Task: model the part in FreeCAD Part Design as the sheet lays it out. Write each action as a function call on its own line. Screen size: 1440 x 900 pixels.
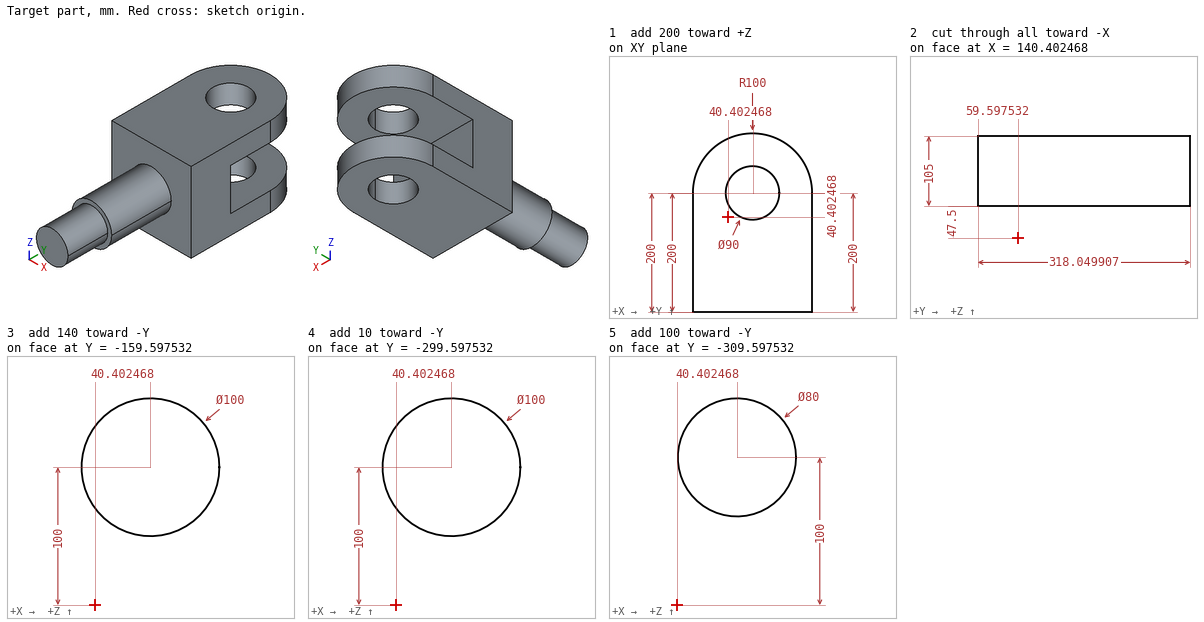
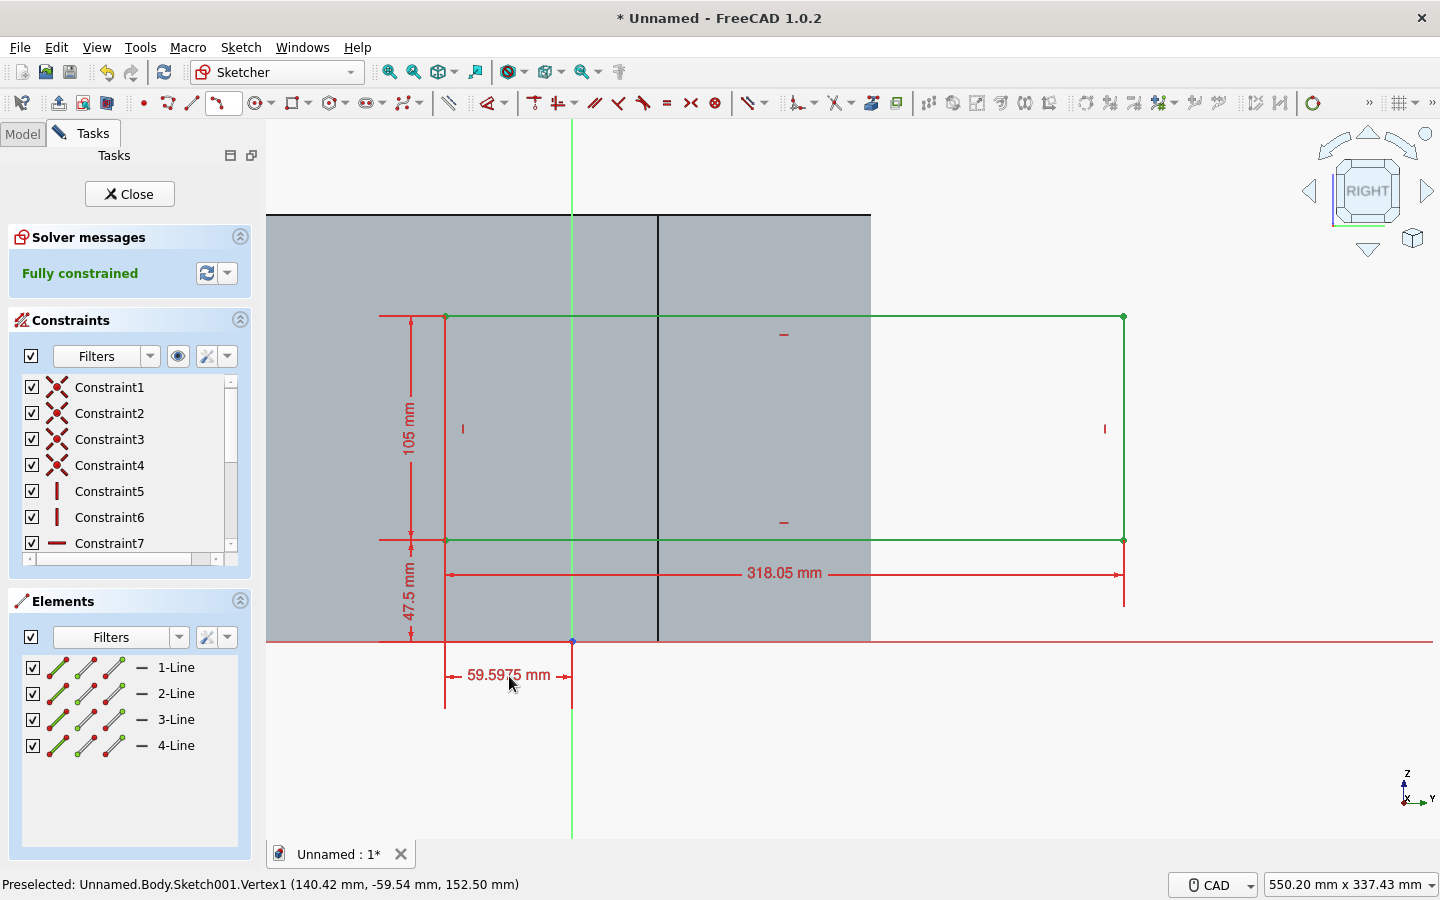
click(130, 194)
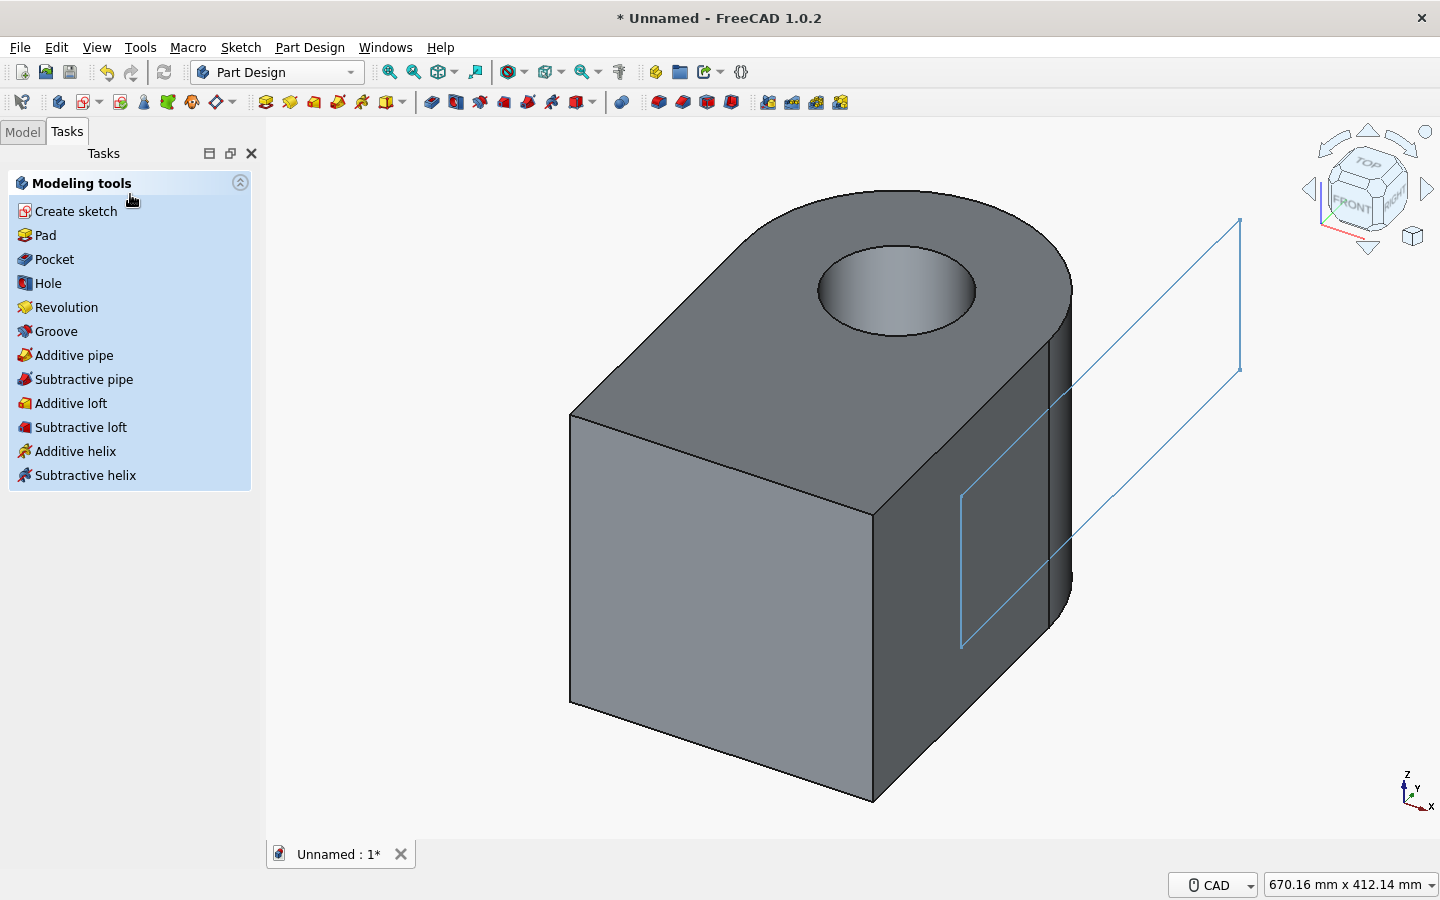
click(432, 102)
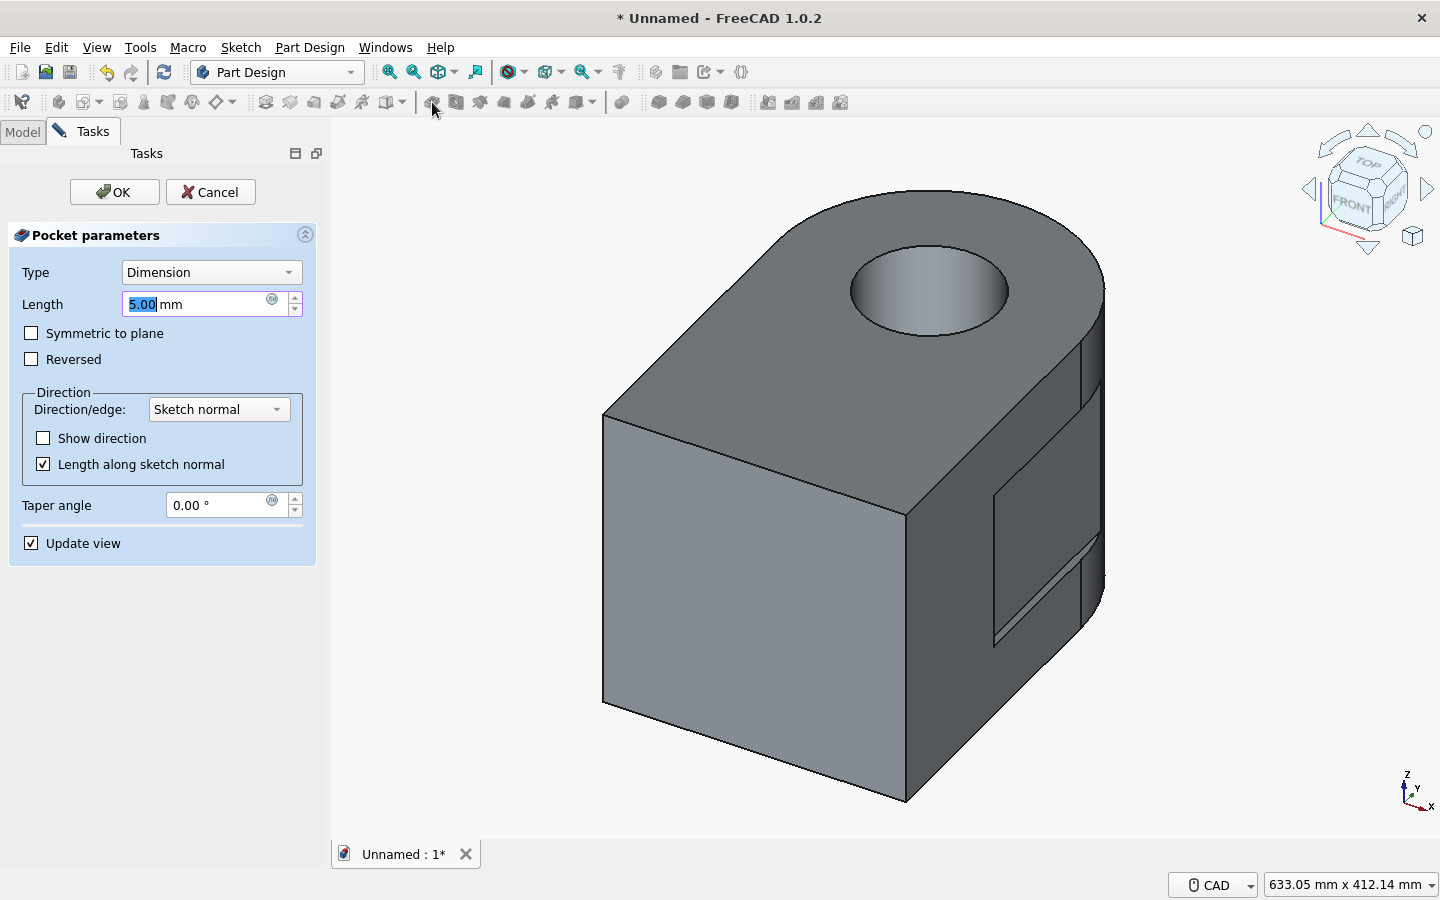
click(212, 272)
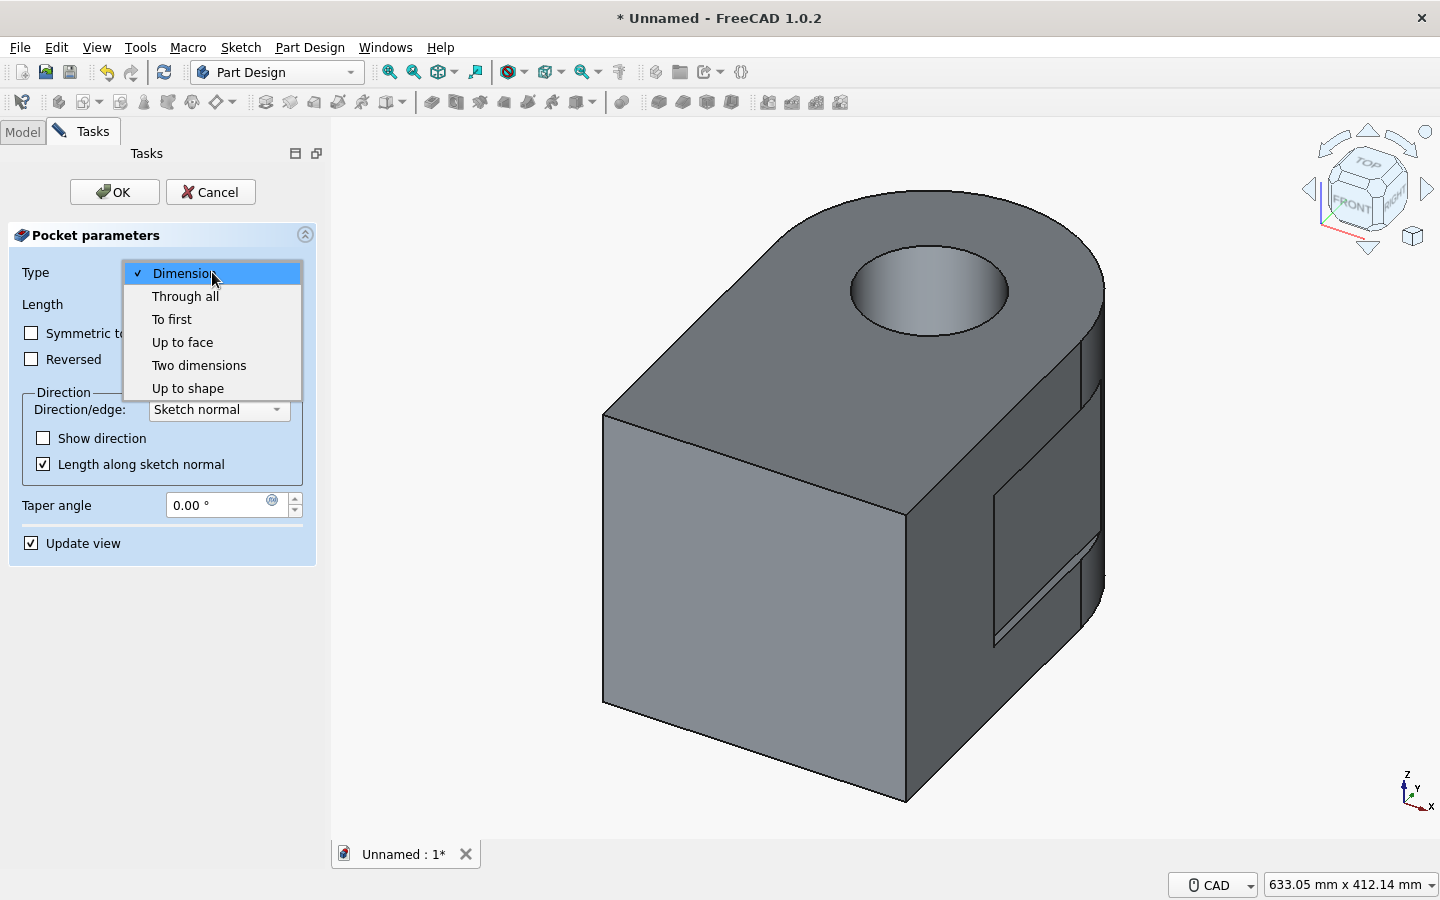
click(212, 296)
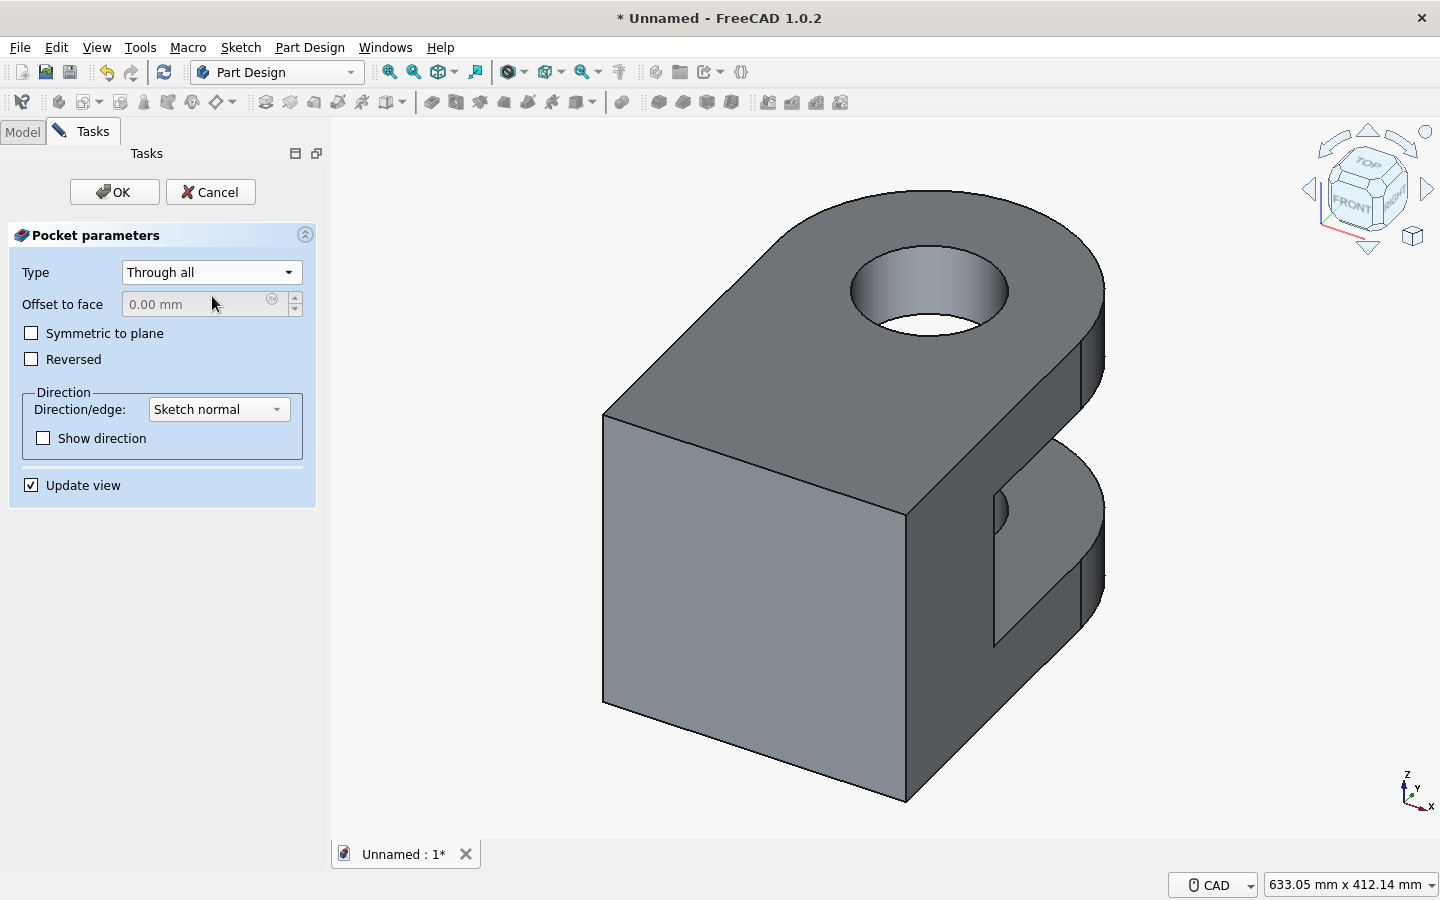
click(115, 192)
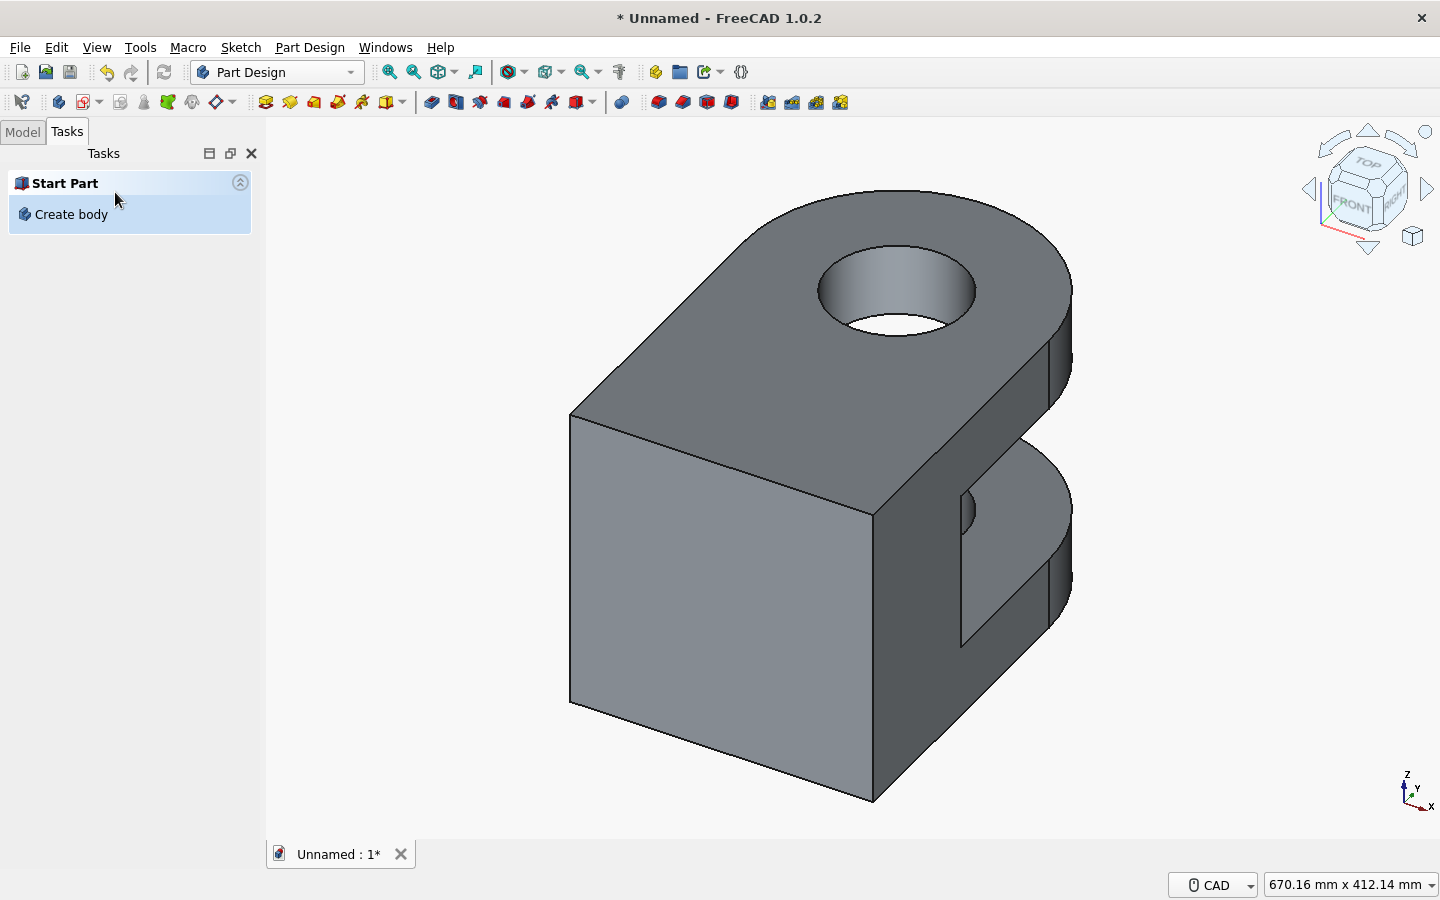
click(722, 607)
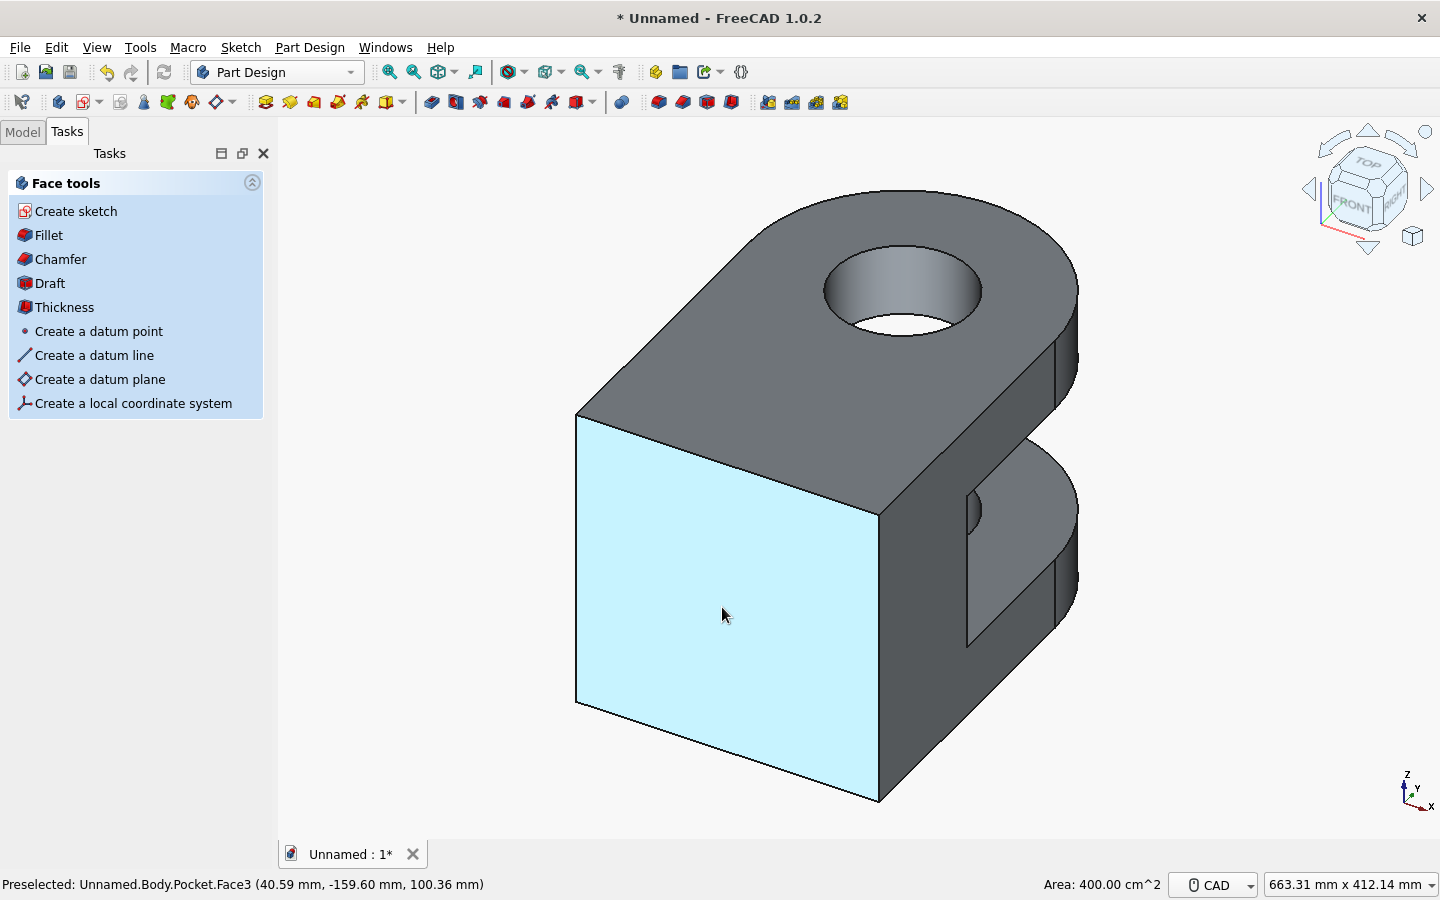
click(84, 102)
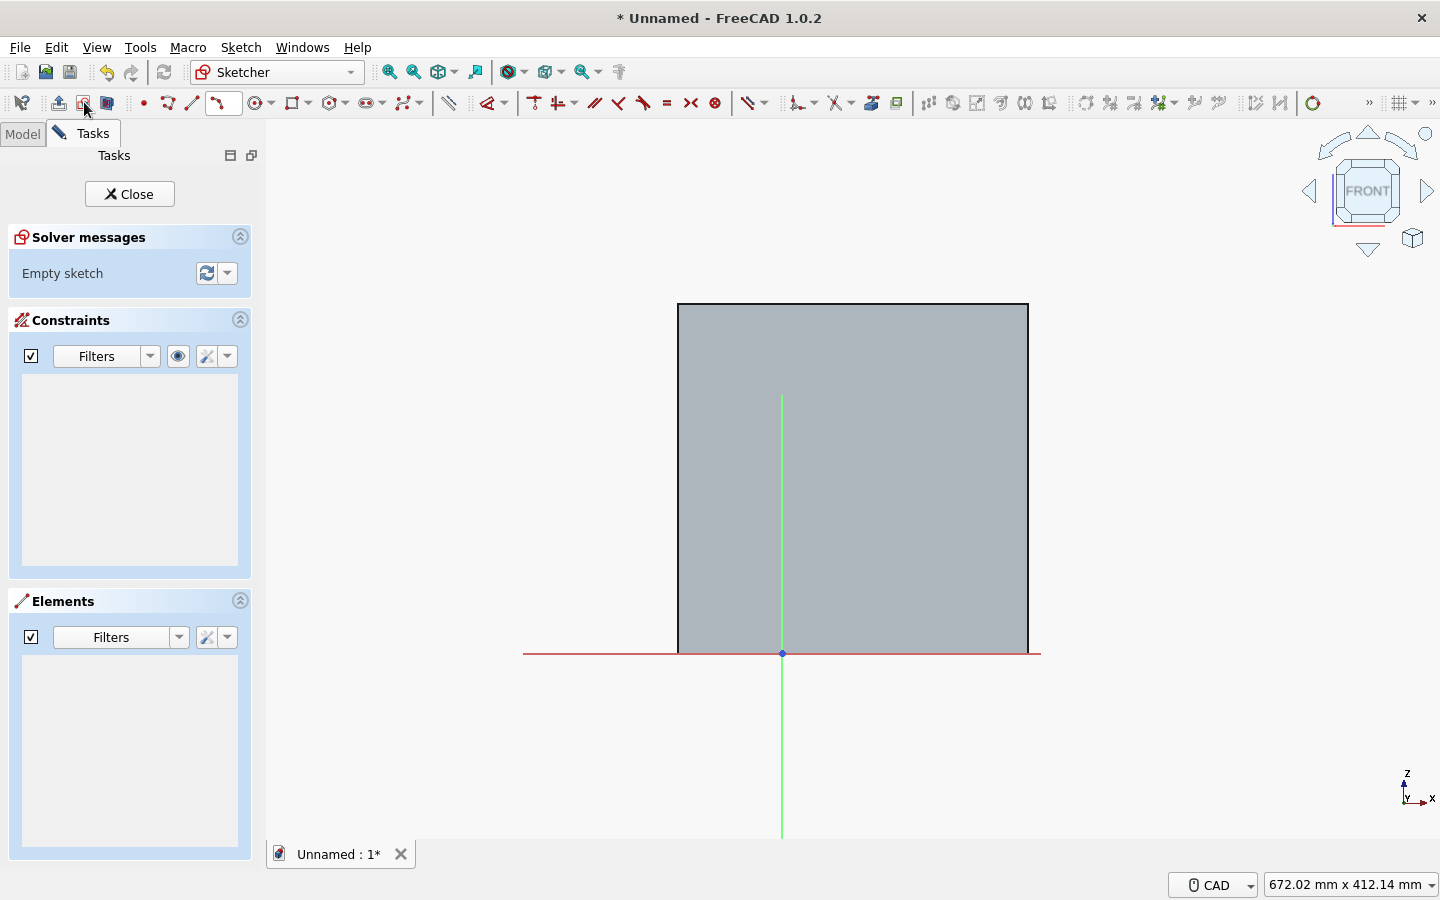
scroll(936, 576, up, 3)